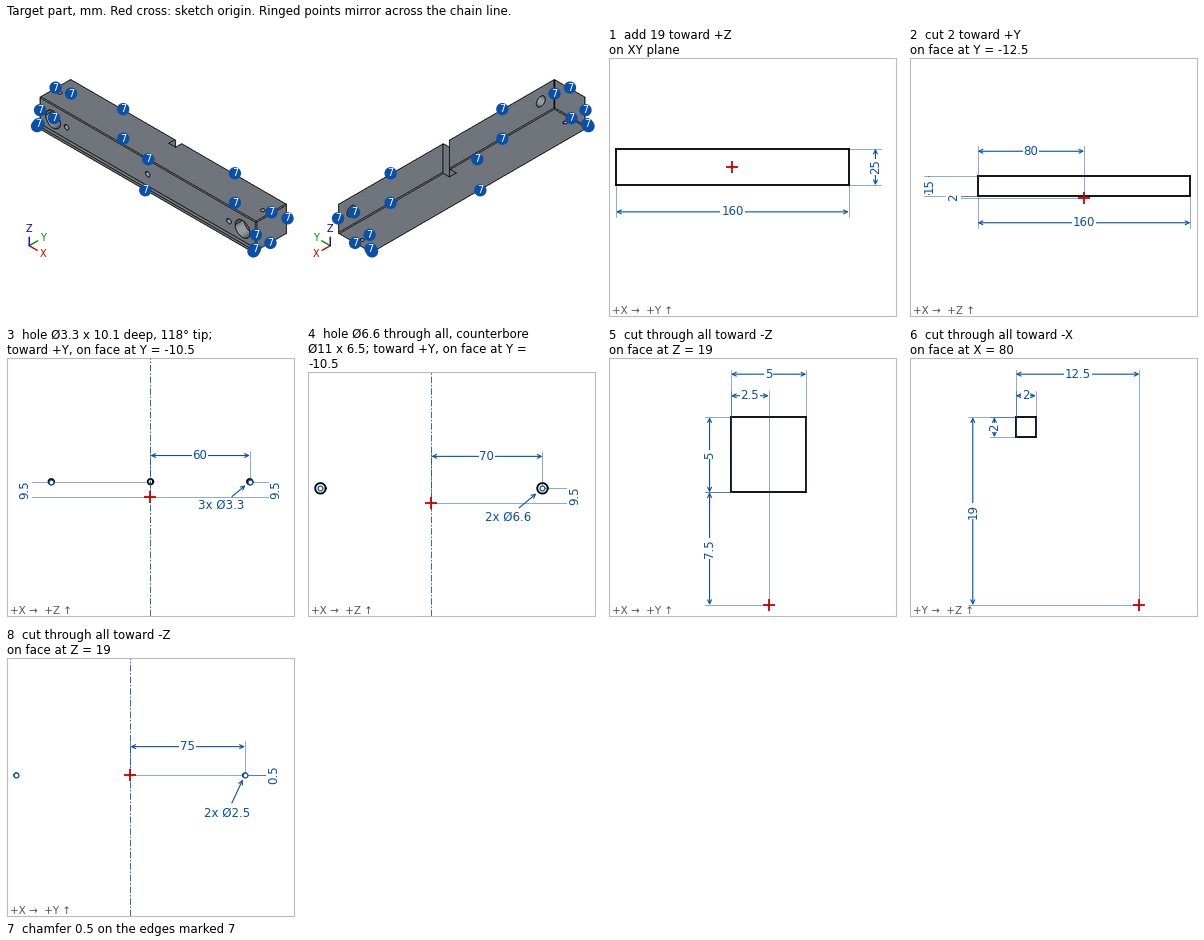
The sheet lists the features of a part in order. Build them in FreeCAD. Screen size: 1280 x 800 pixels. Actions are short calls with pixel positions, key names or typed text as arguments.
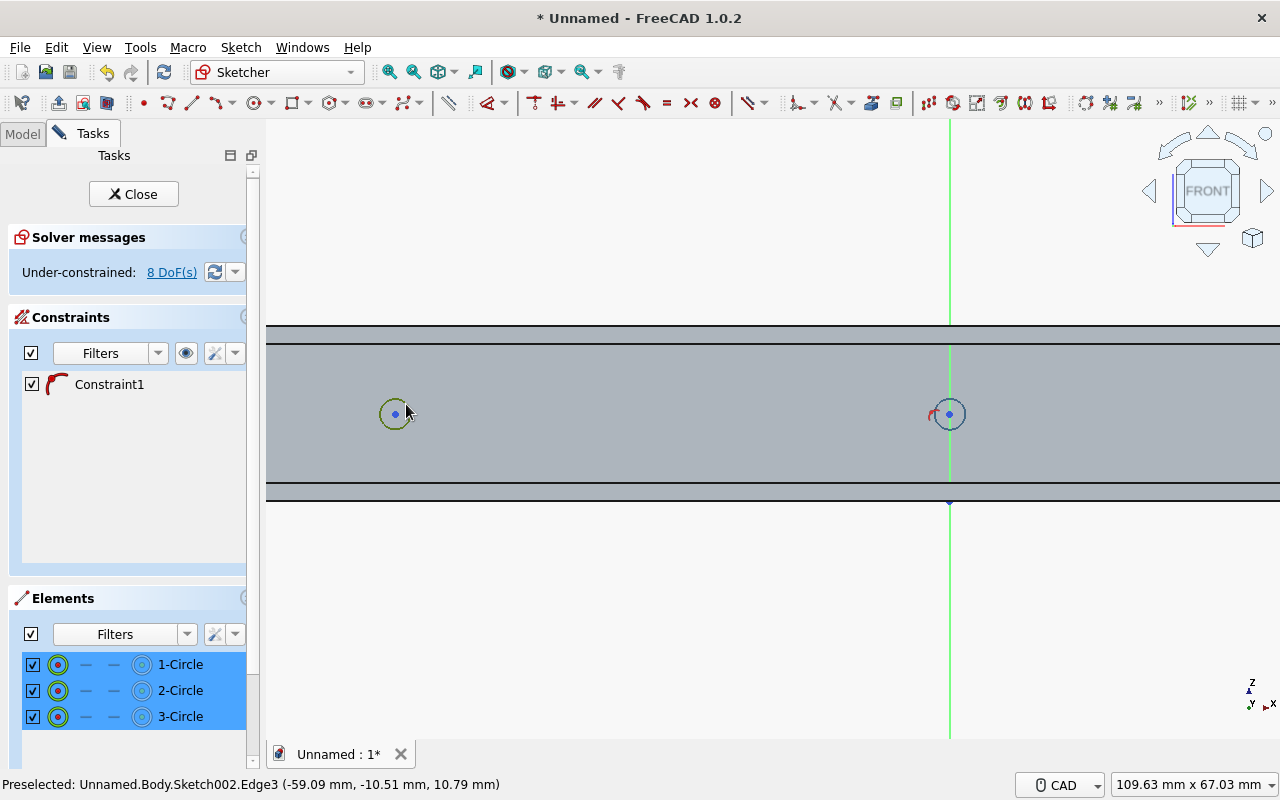
click(668, 104)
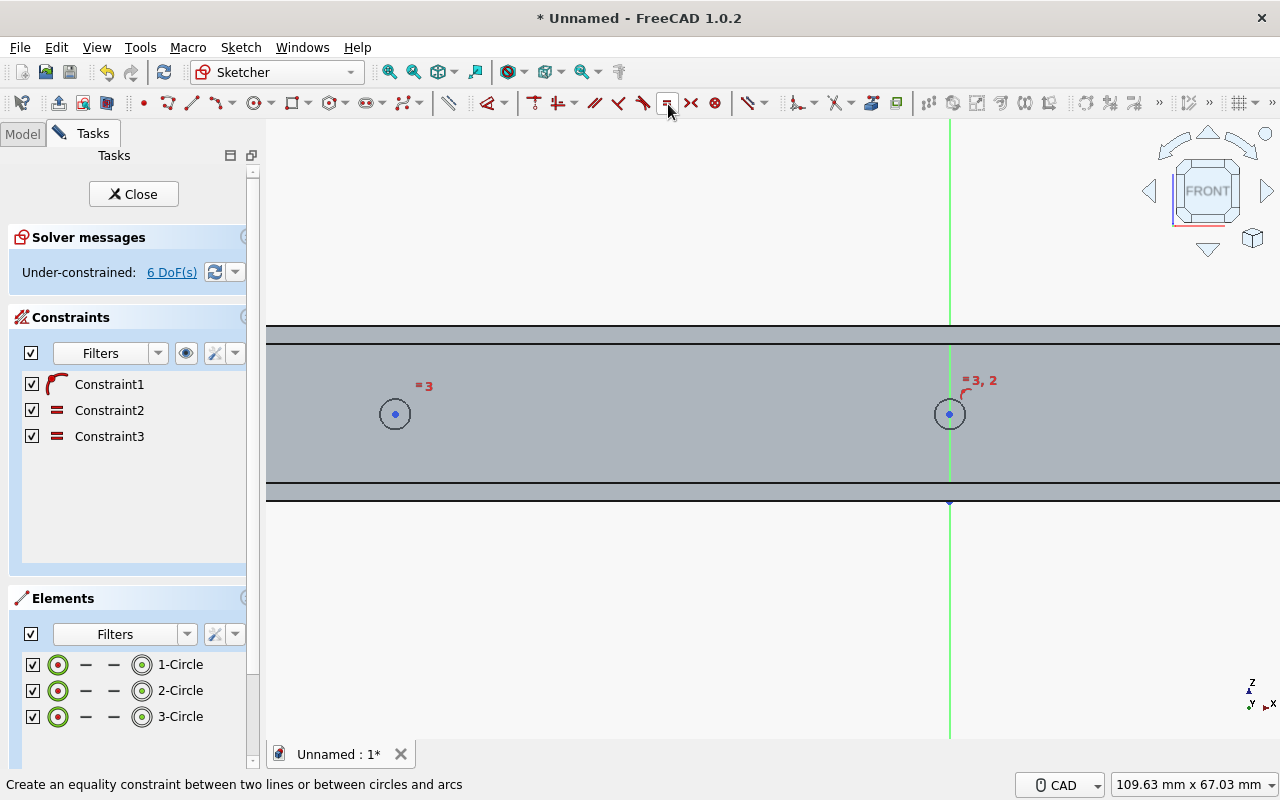
scroll(406, 404, down, 3)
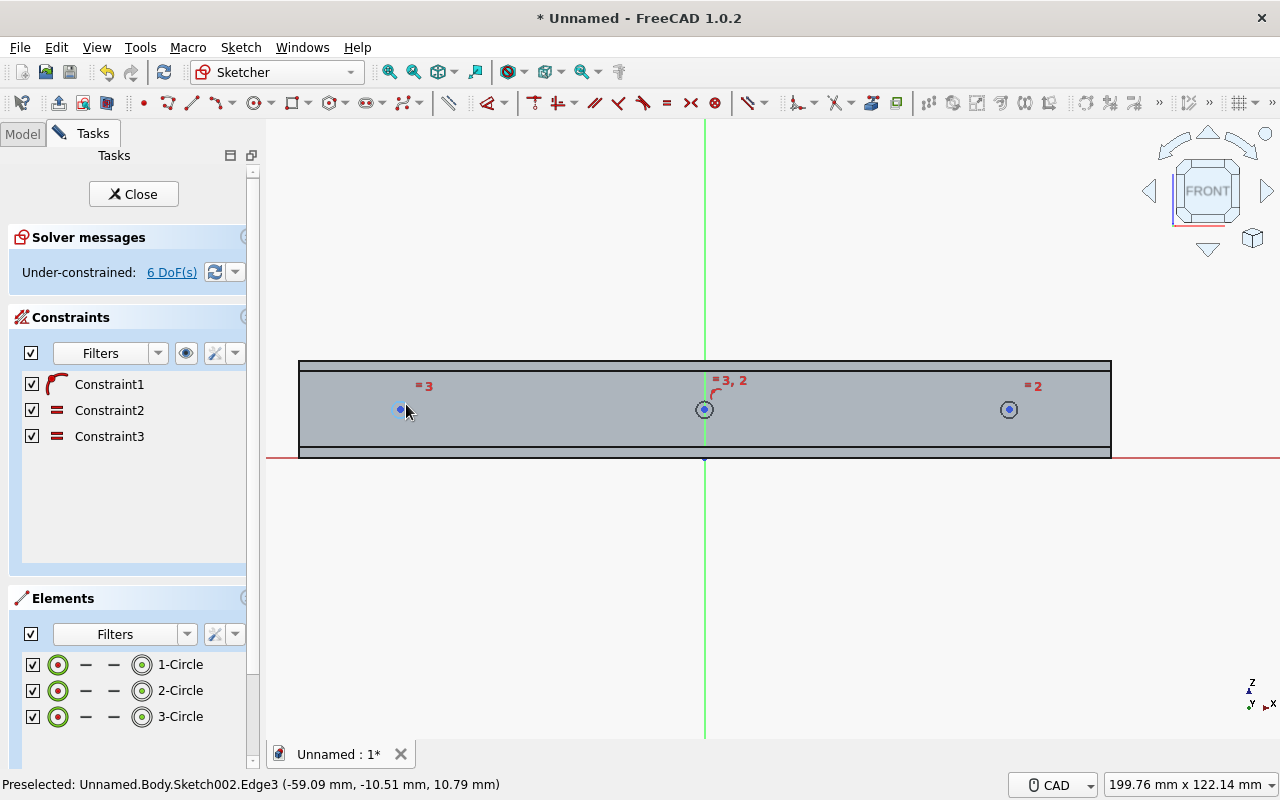
click(1009, 410)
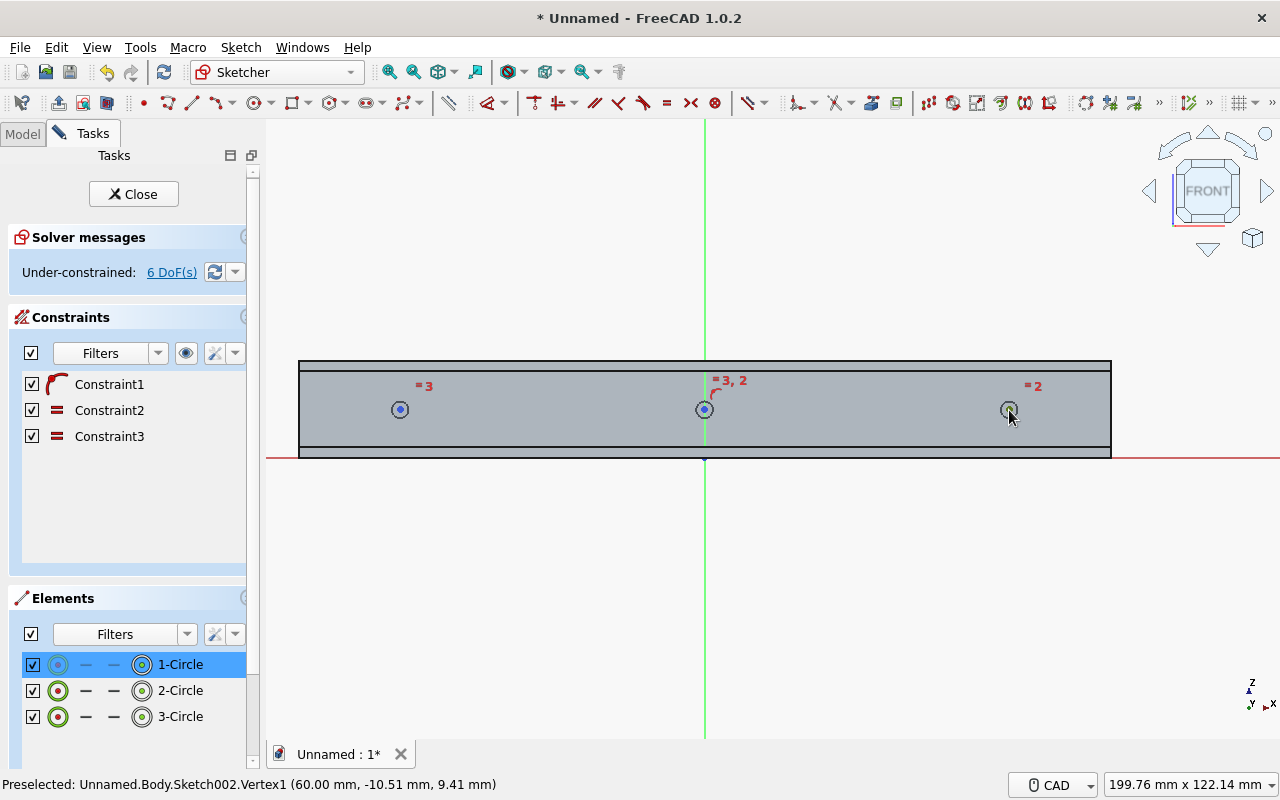
click(400, 410)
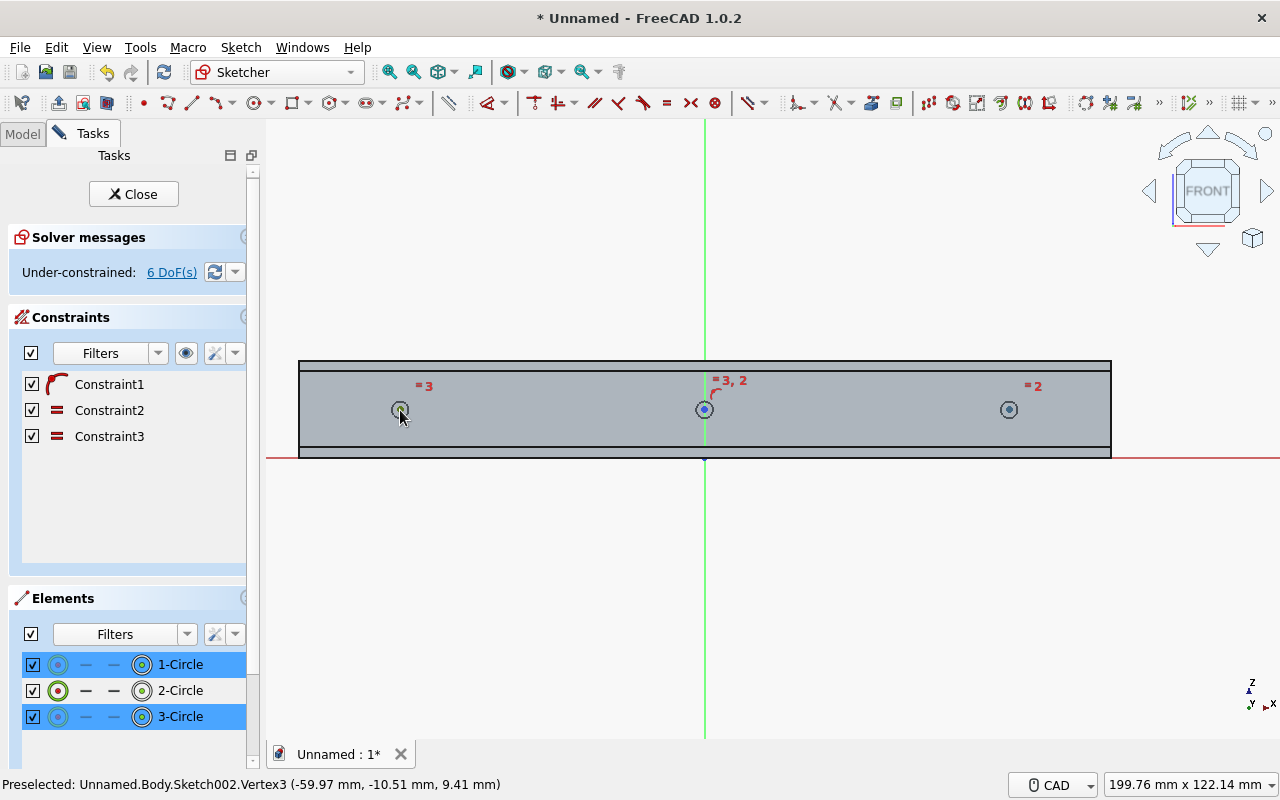
click(705, 671)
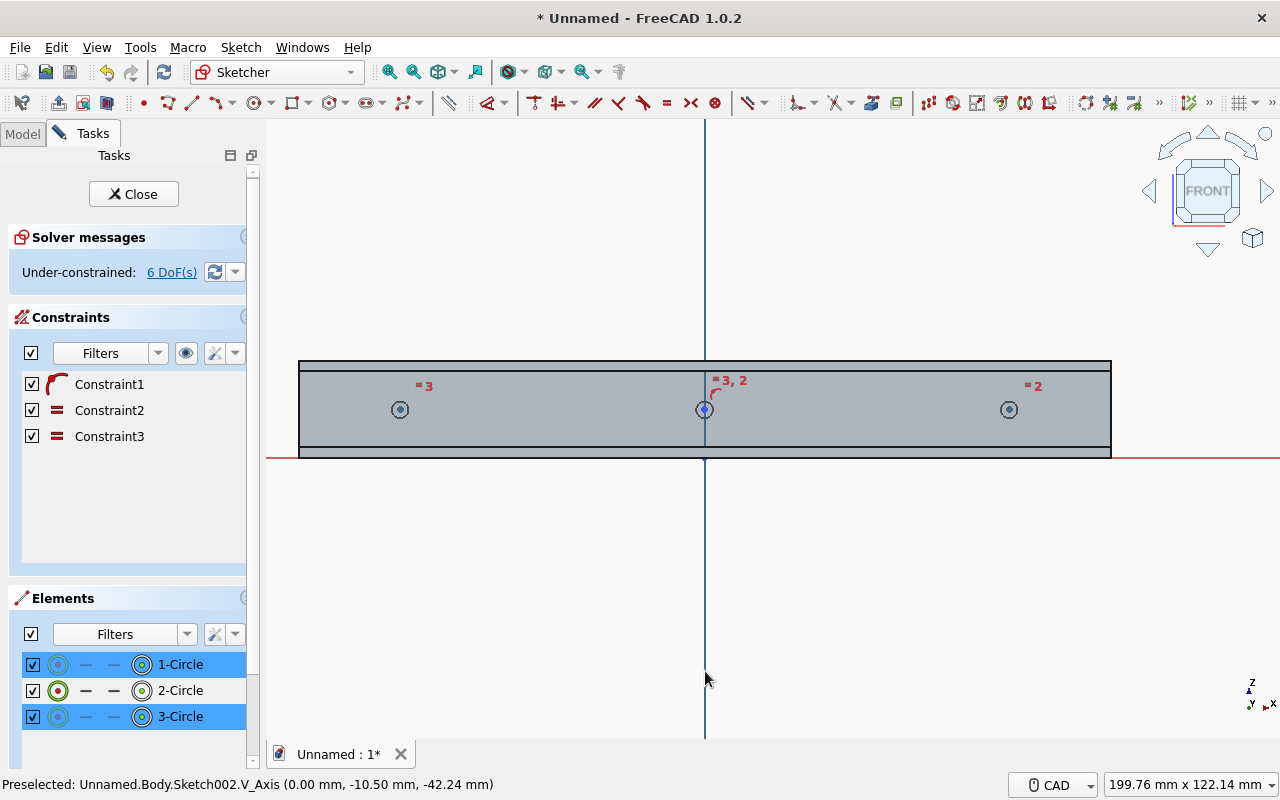
click(692, 104)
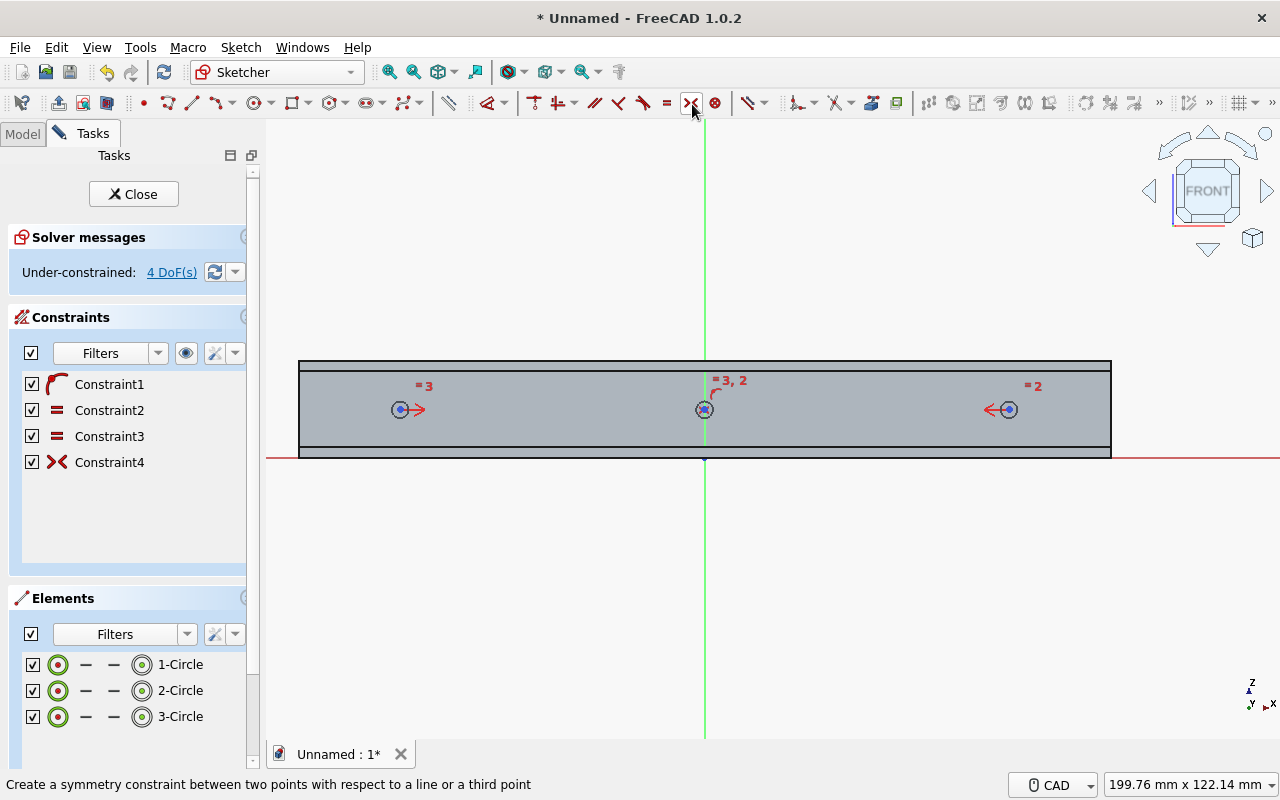
click(488, 104)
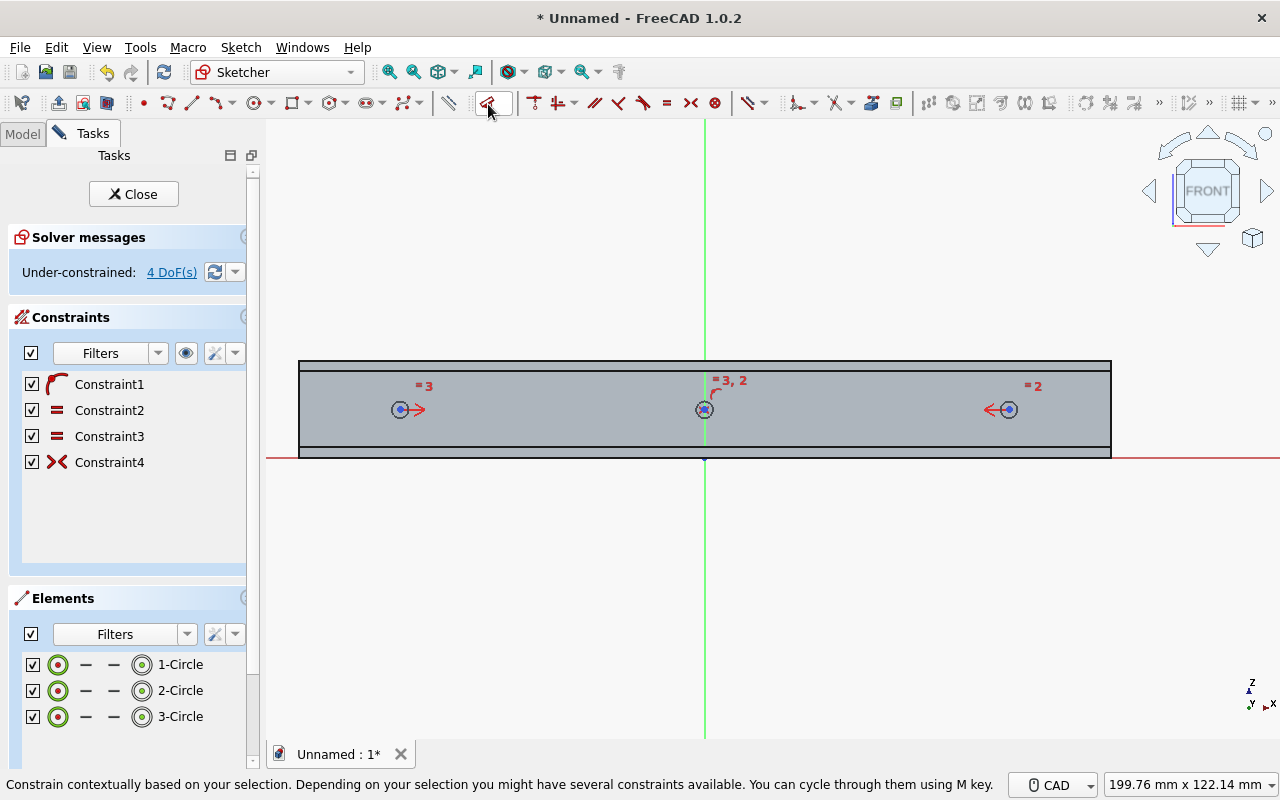
scroll(1015, 416, up, 5)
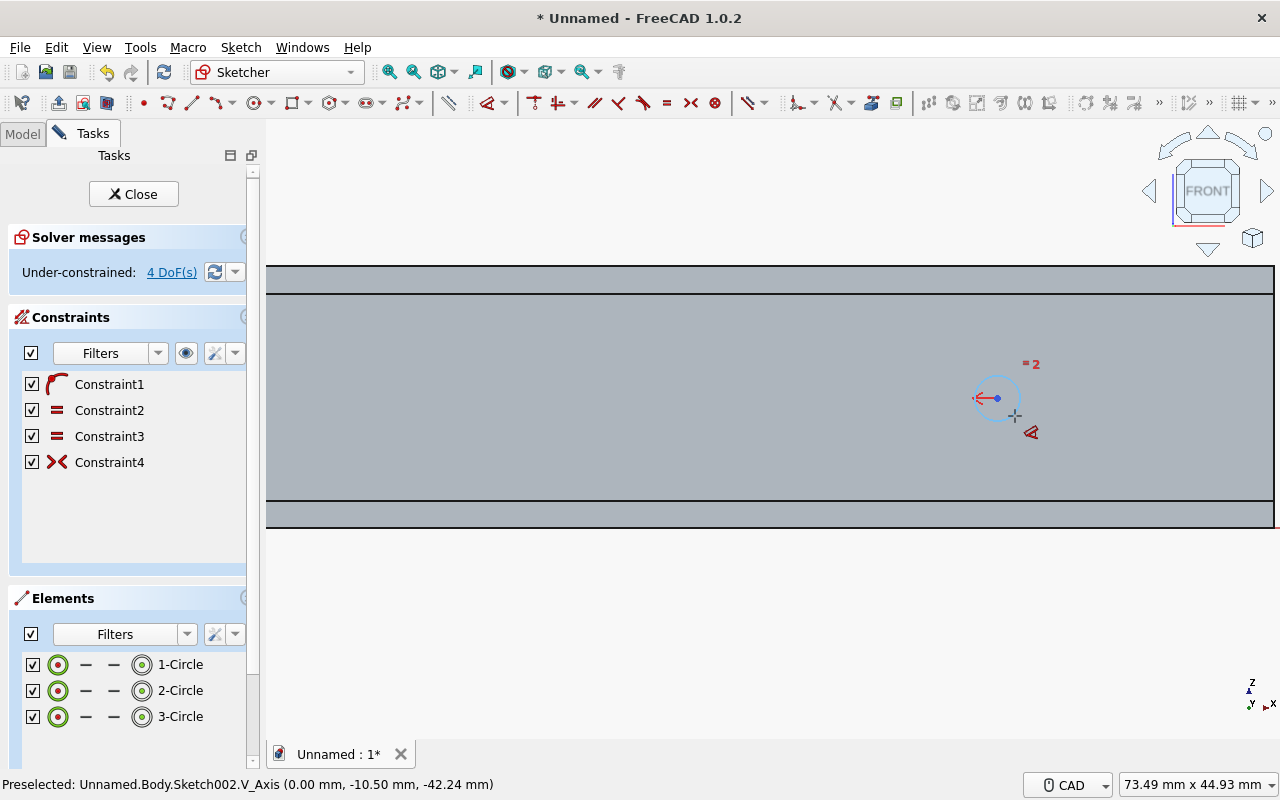
click(1014, 414)
click(1037, 436)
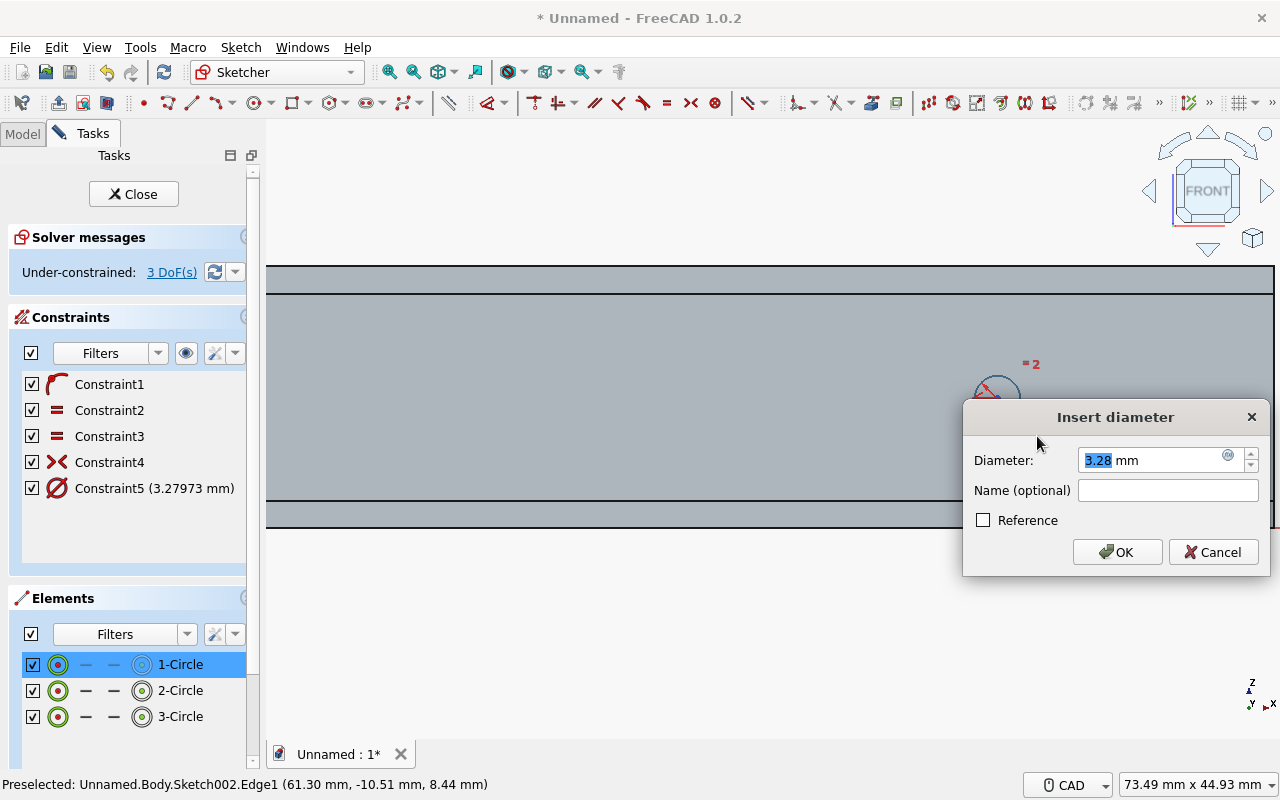
text(3.3)
key(Return)